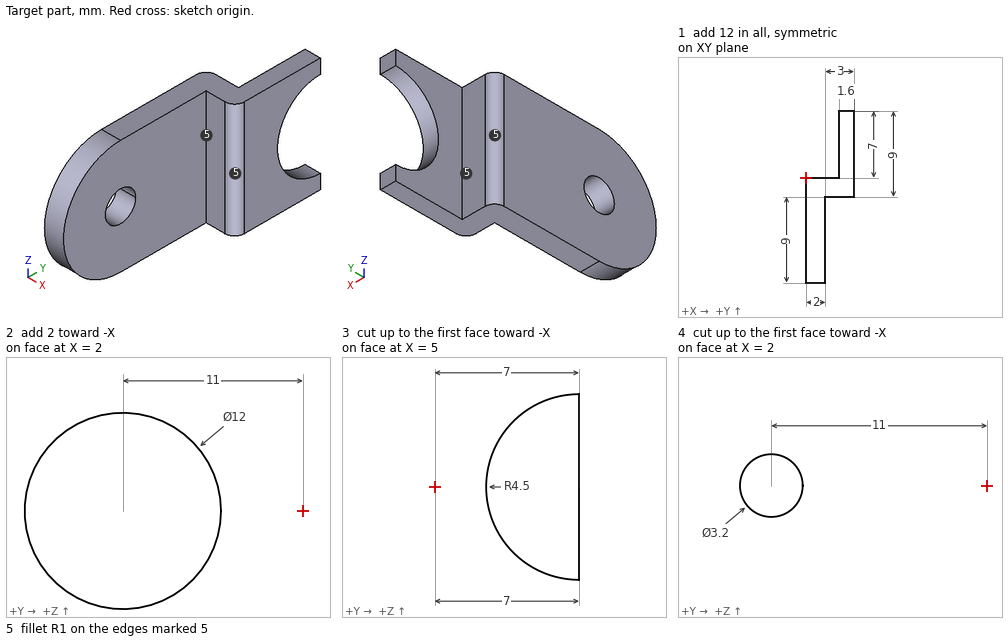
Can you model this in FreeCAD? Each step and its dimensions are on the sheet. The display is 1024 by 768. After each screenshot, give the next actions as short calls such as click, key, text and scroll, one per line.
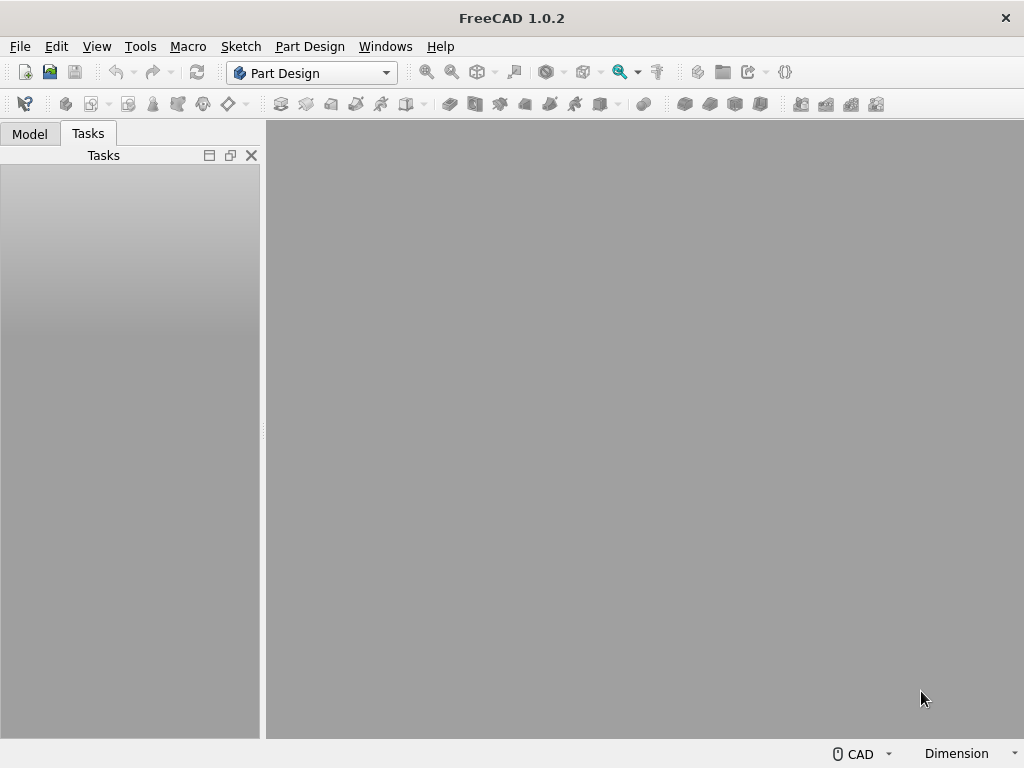
key(ctrl+n)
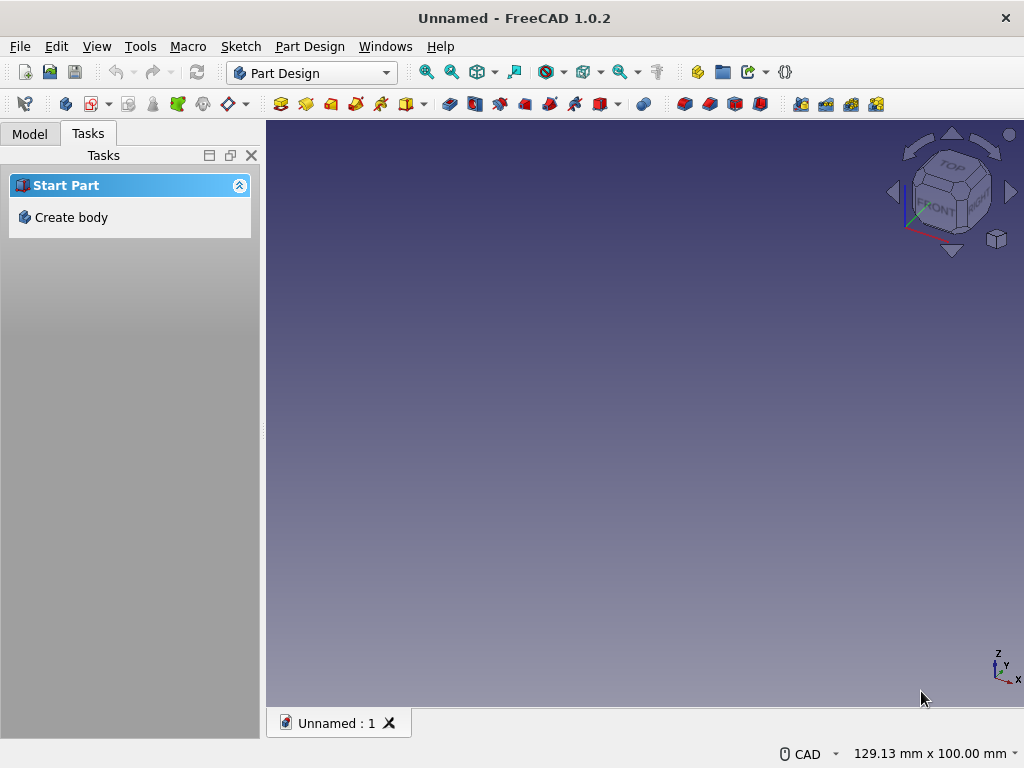
click(90, 104)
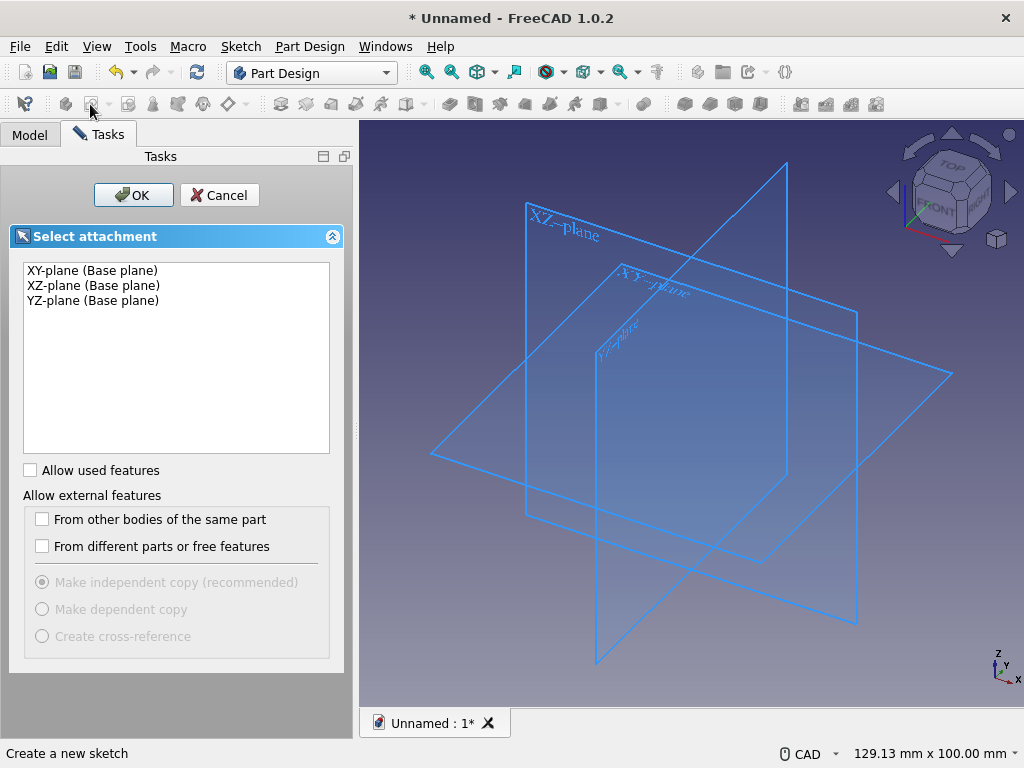
click(84, 270)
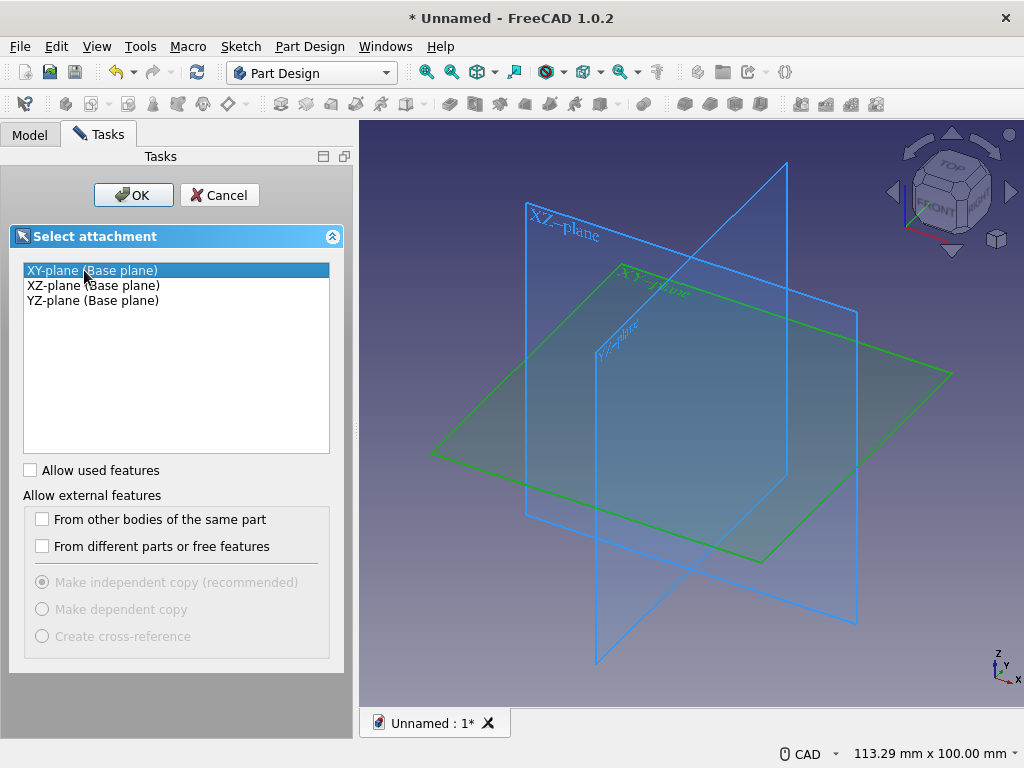
click(134, 195)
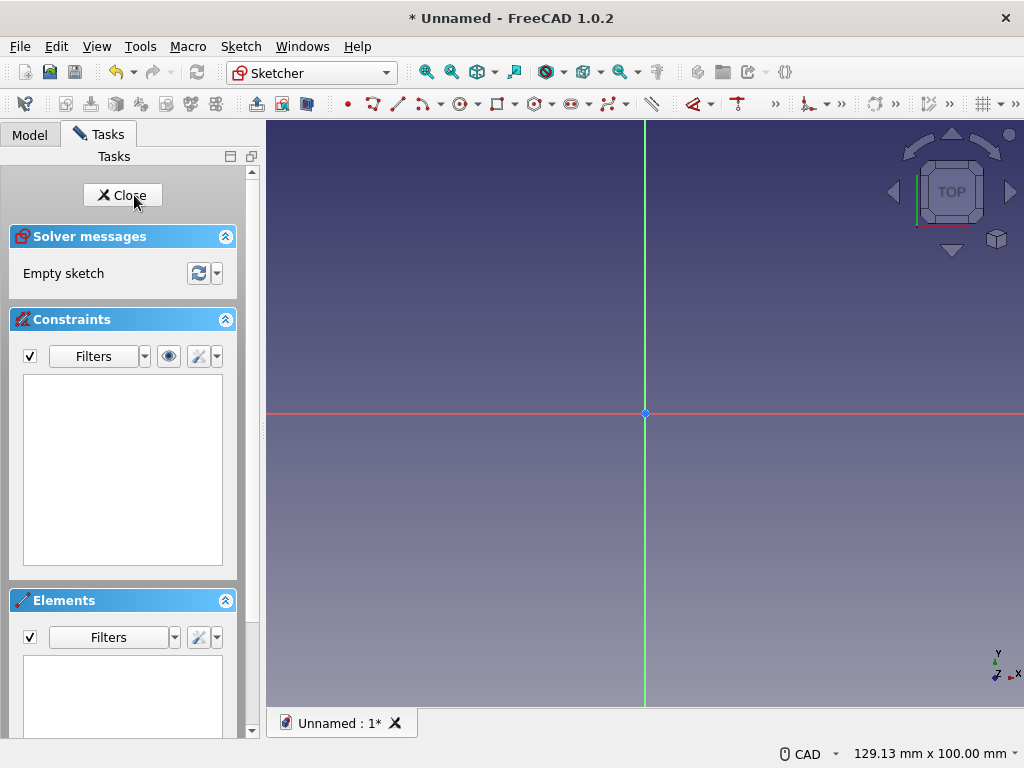
scroll(696, 430, up, 6)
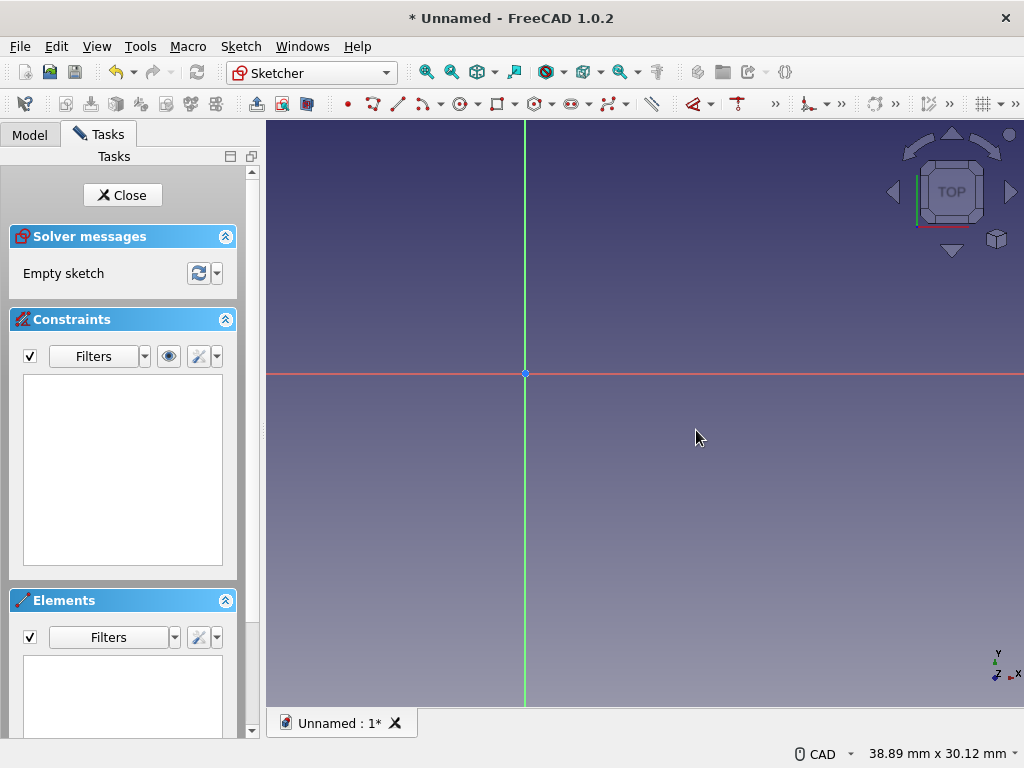
key(g)
key(m)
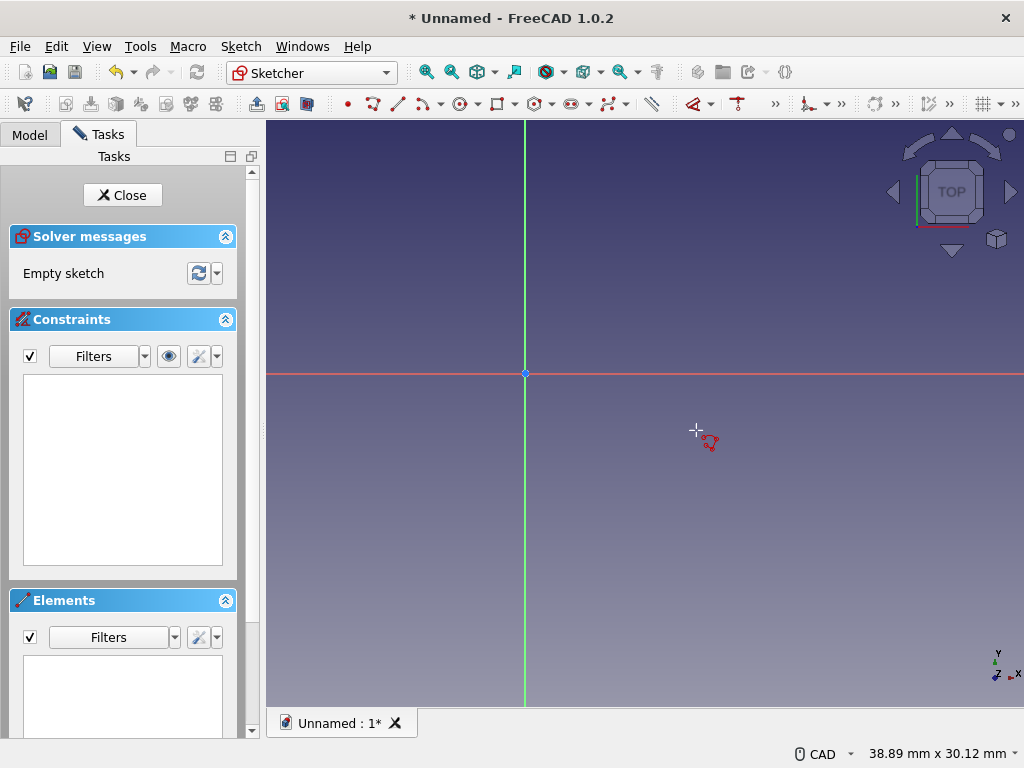
click(525, 374)
click(534, 588)
click(564, 588)
click(564, 413)
click(623, 413)
click(623, 238)
click(592, 238)
click(592, 383)
click(525, 374)
key(Escape)
key(Escape)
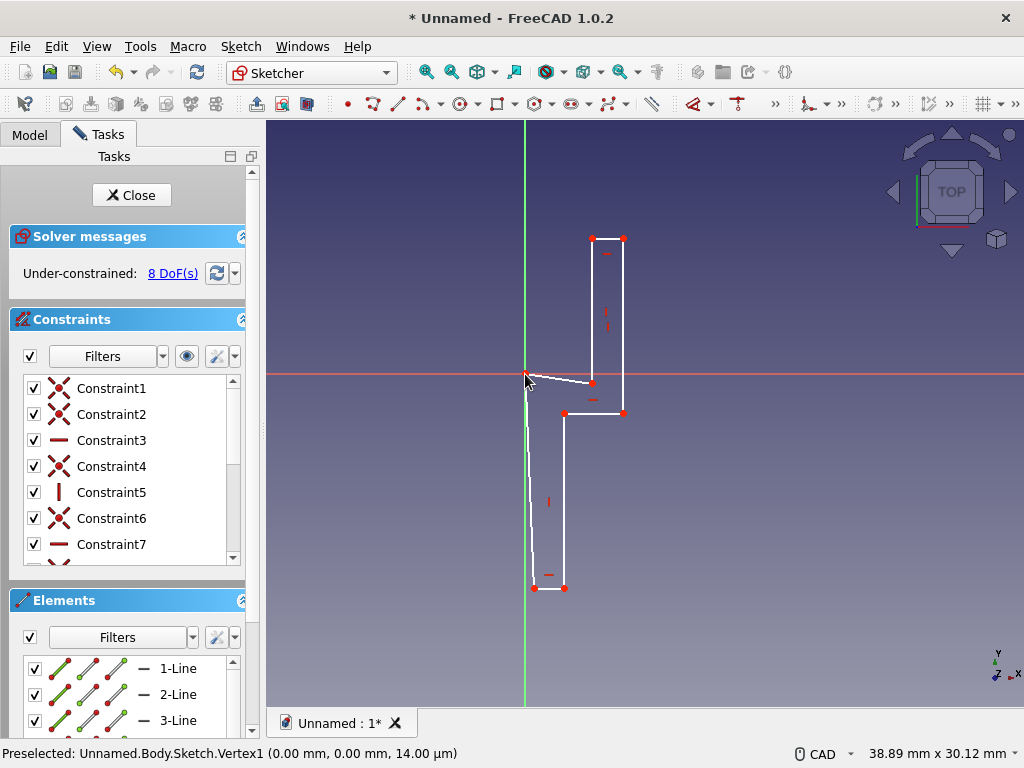
click(528, 438)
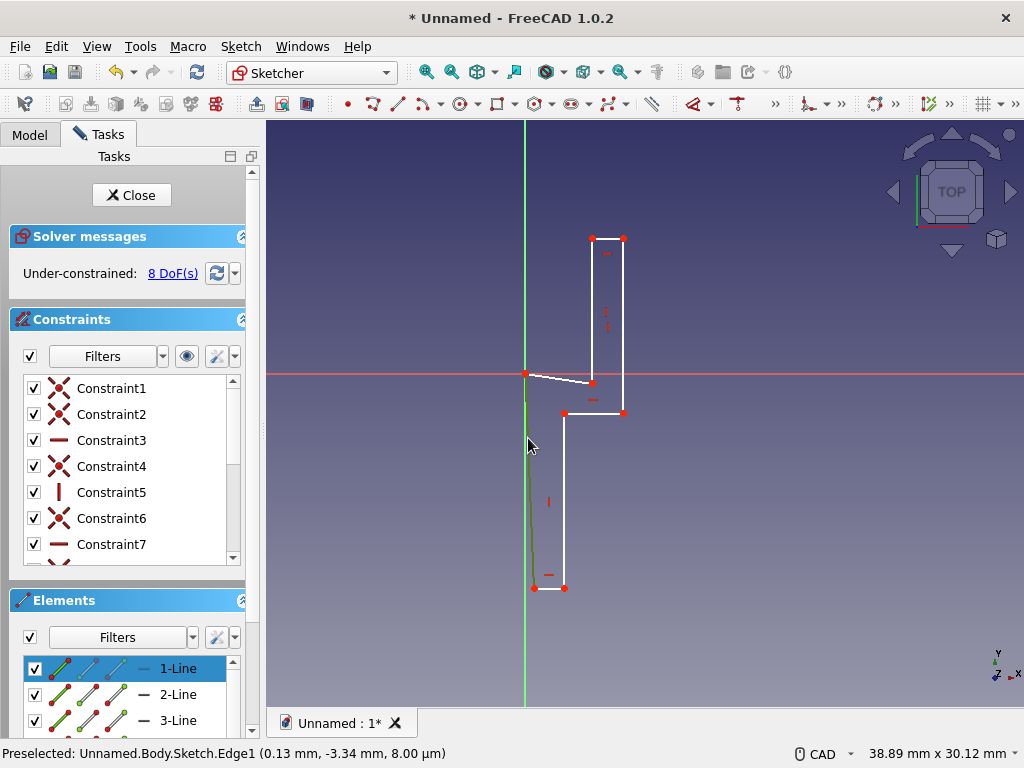
key(v)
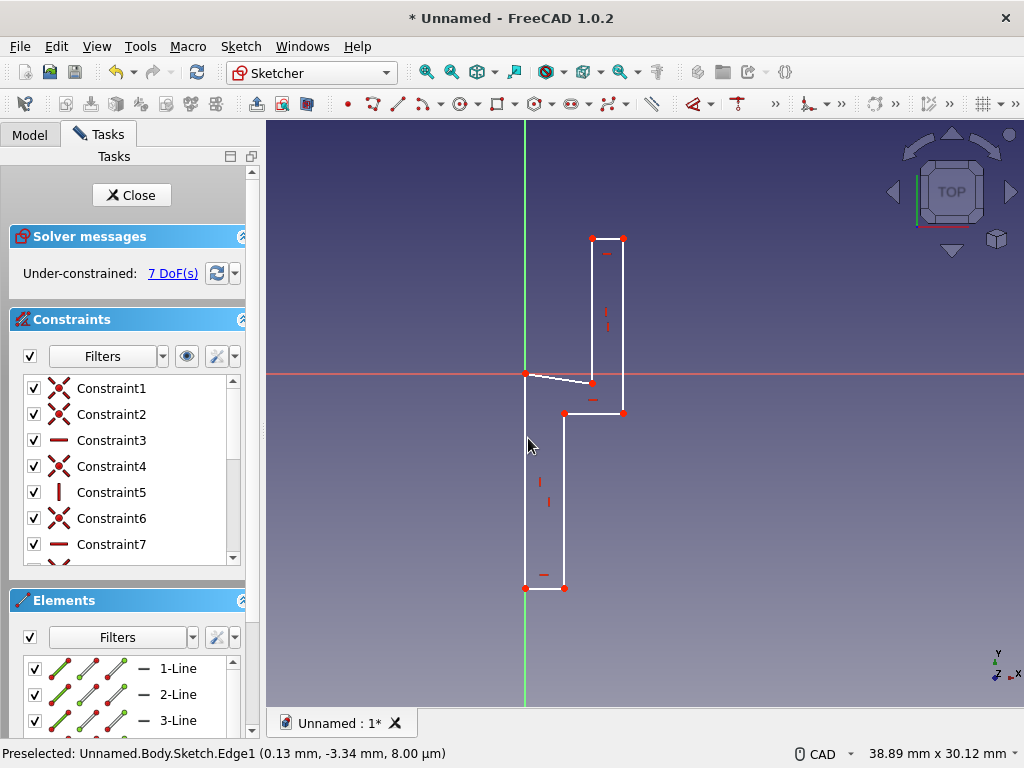
click(545, 377)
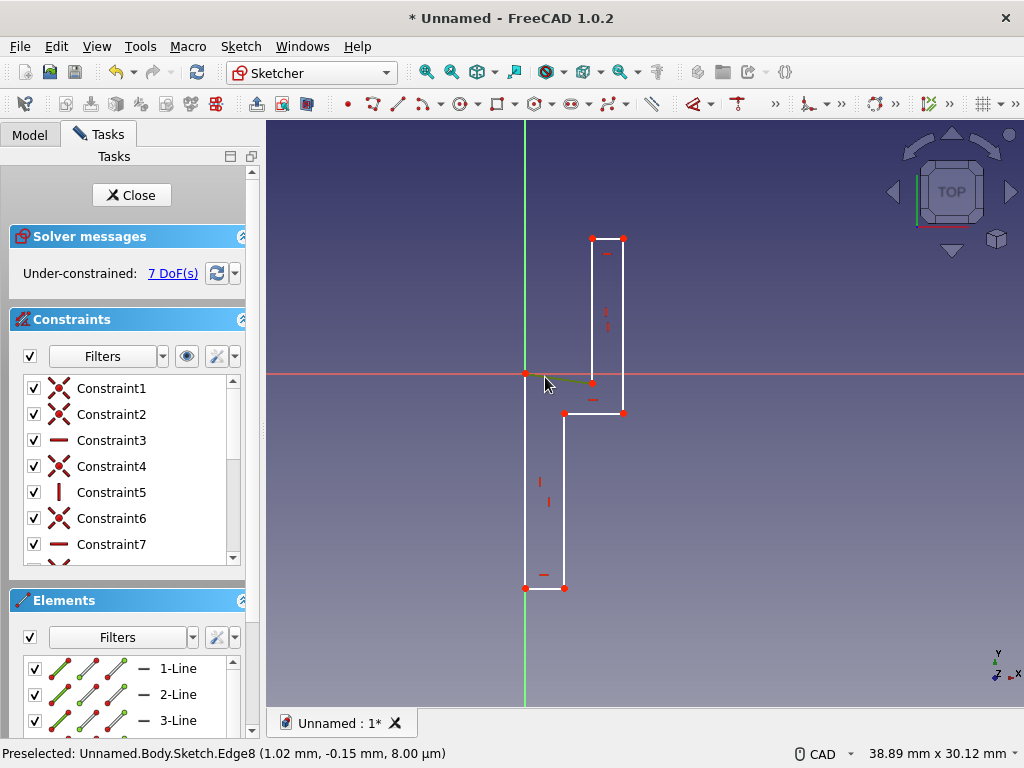
key(h)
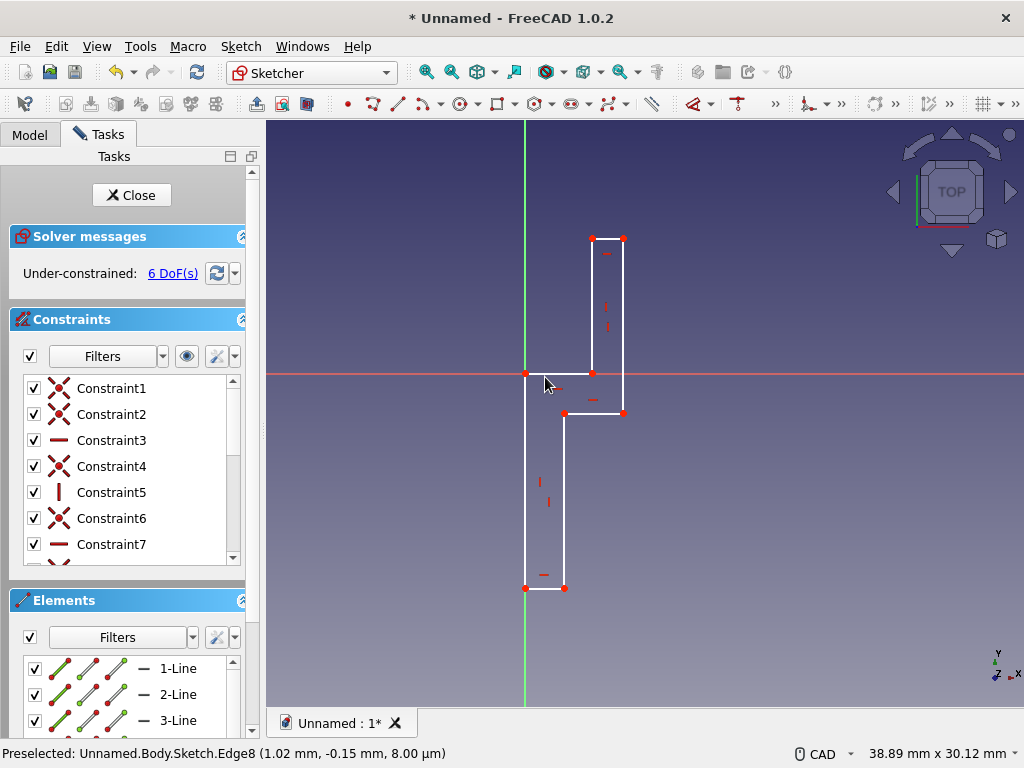
key(d)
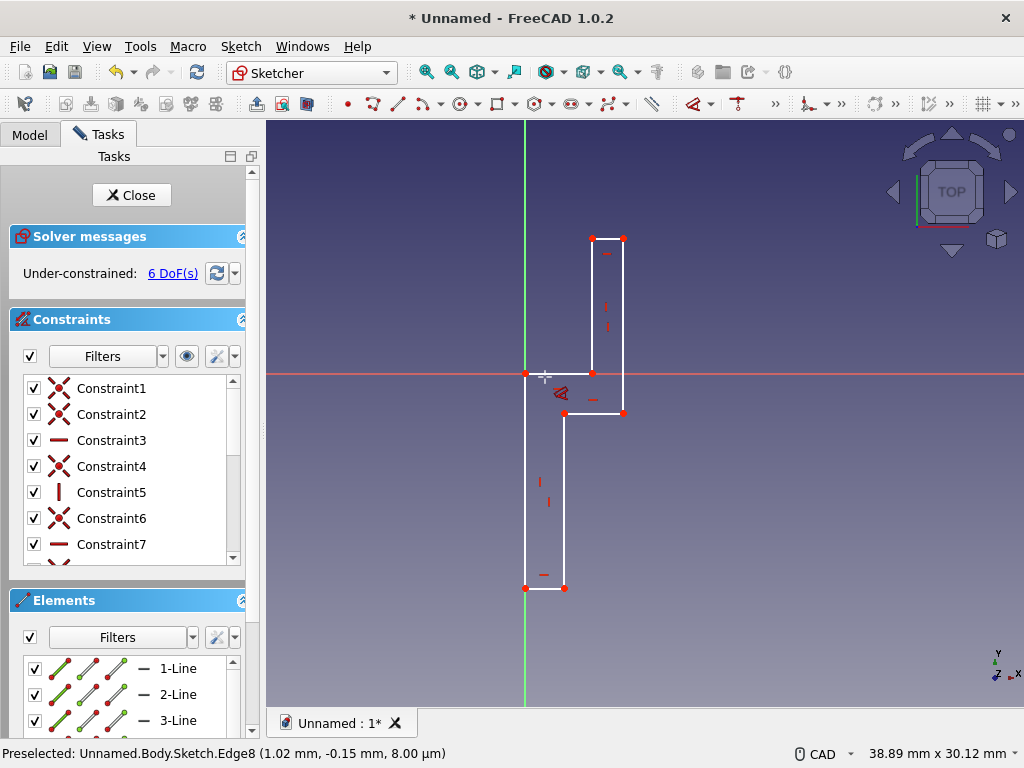
click(537, 589)
click(545, 623)